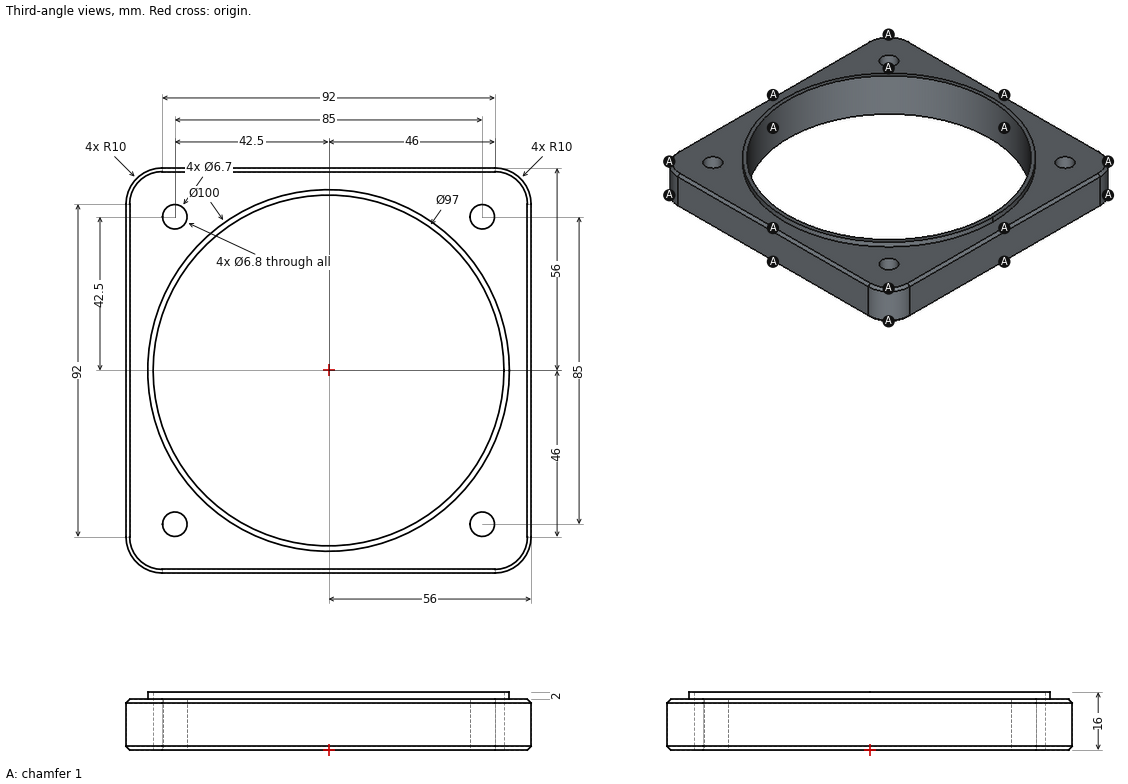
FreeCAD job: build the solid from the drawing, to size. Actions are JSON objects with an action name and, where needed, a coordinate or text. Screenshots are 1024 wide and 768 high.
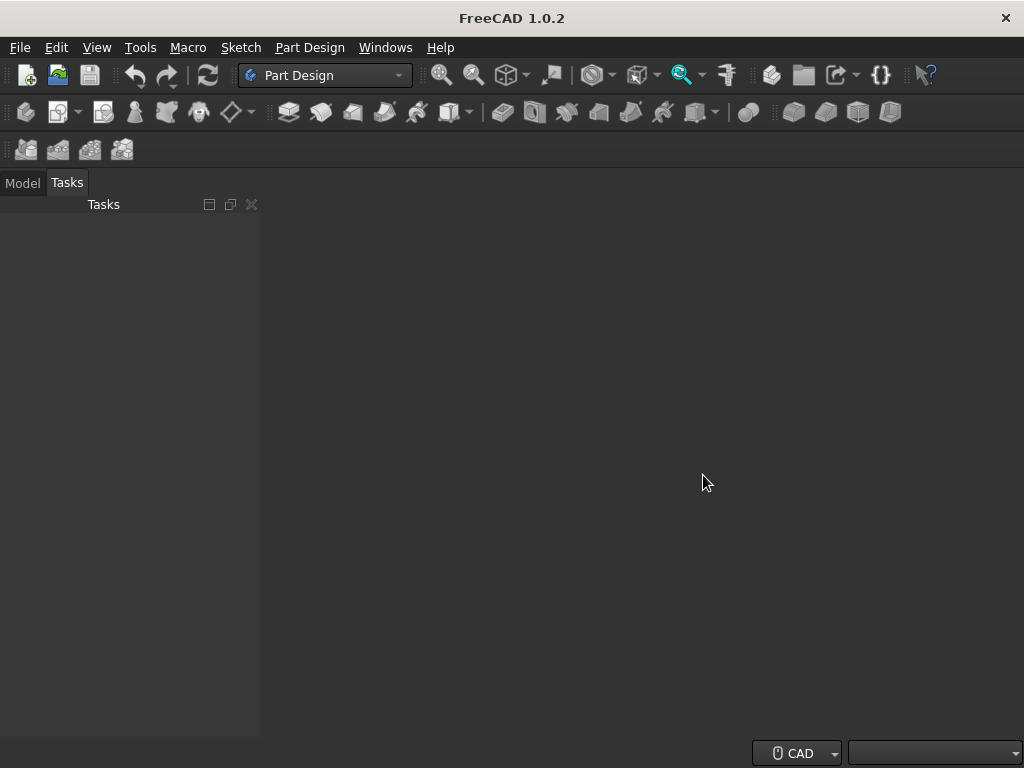
{"action": "left_click", "coordinate": [26, 76]}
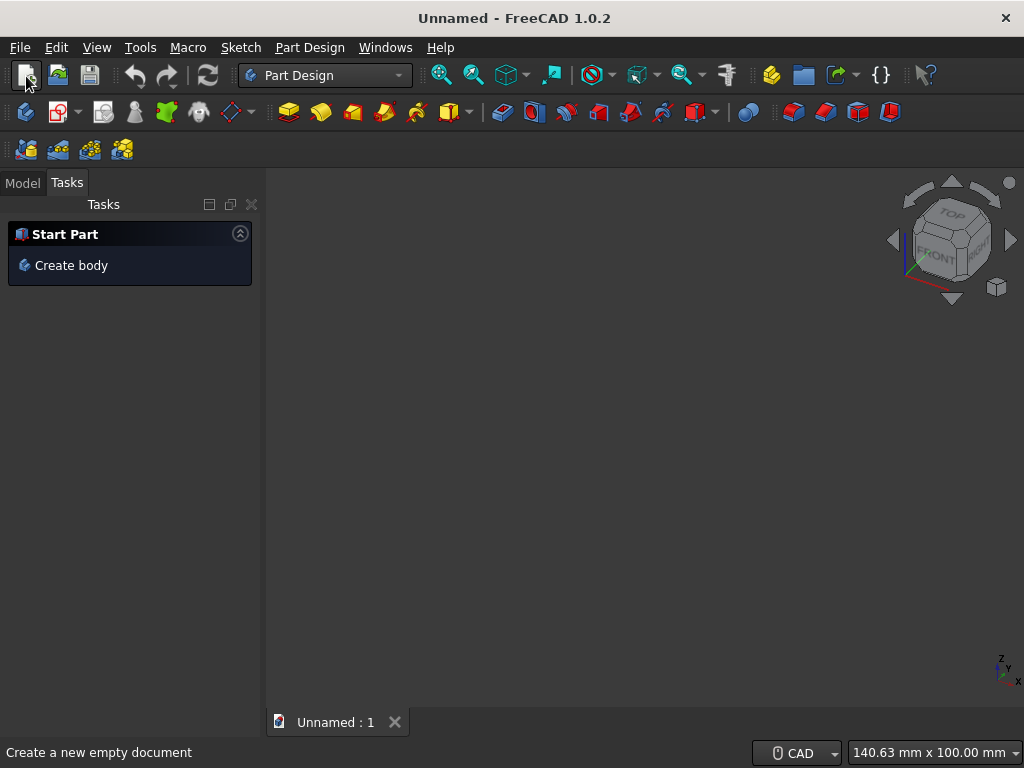
{"action": "left_click", "coordinate": [58, 112]}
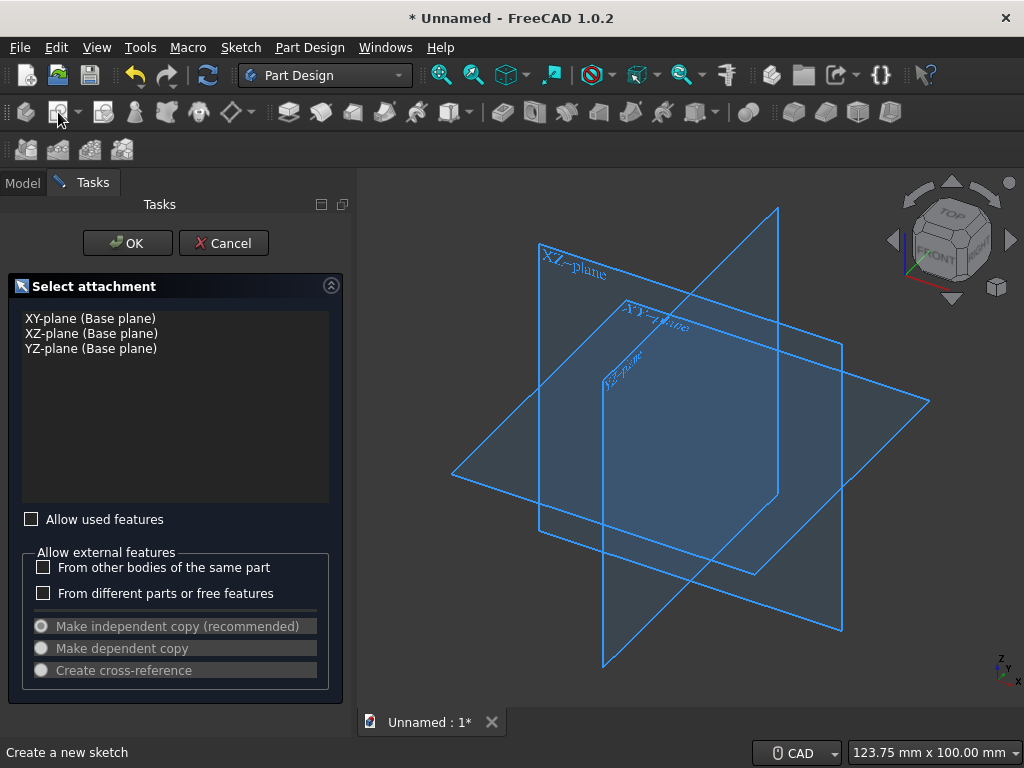
{"action": "left_click", "coordinate": [82, 318]}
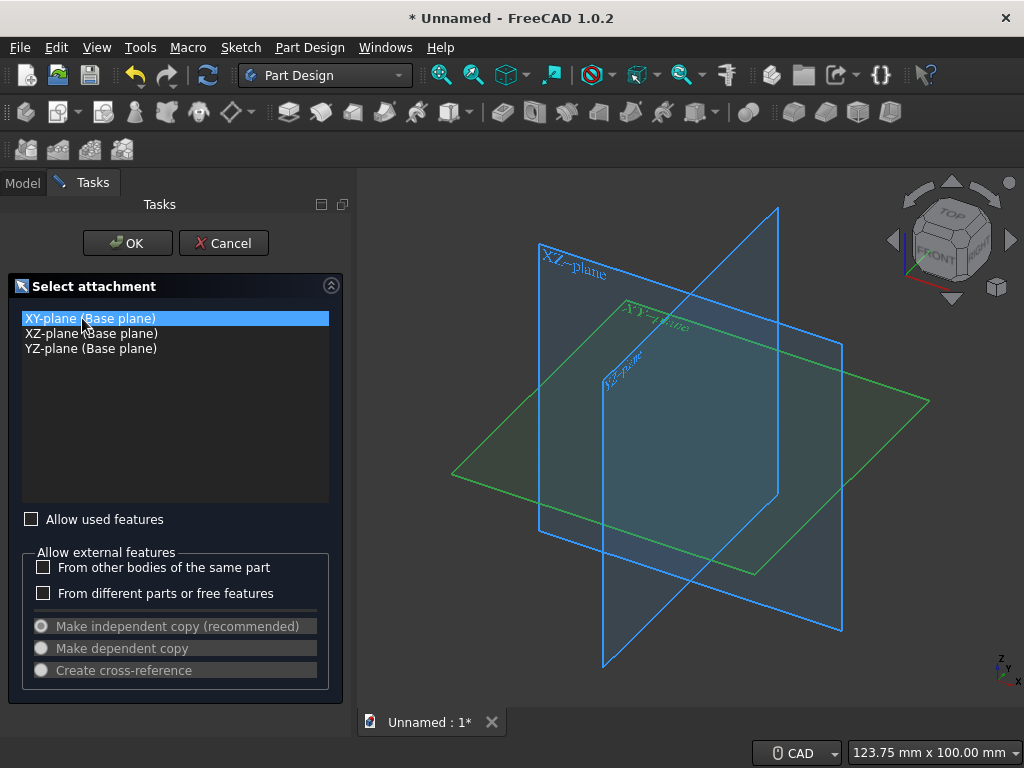
{"action": "left_click", "coordinate": [128, 243]}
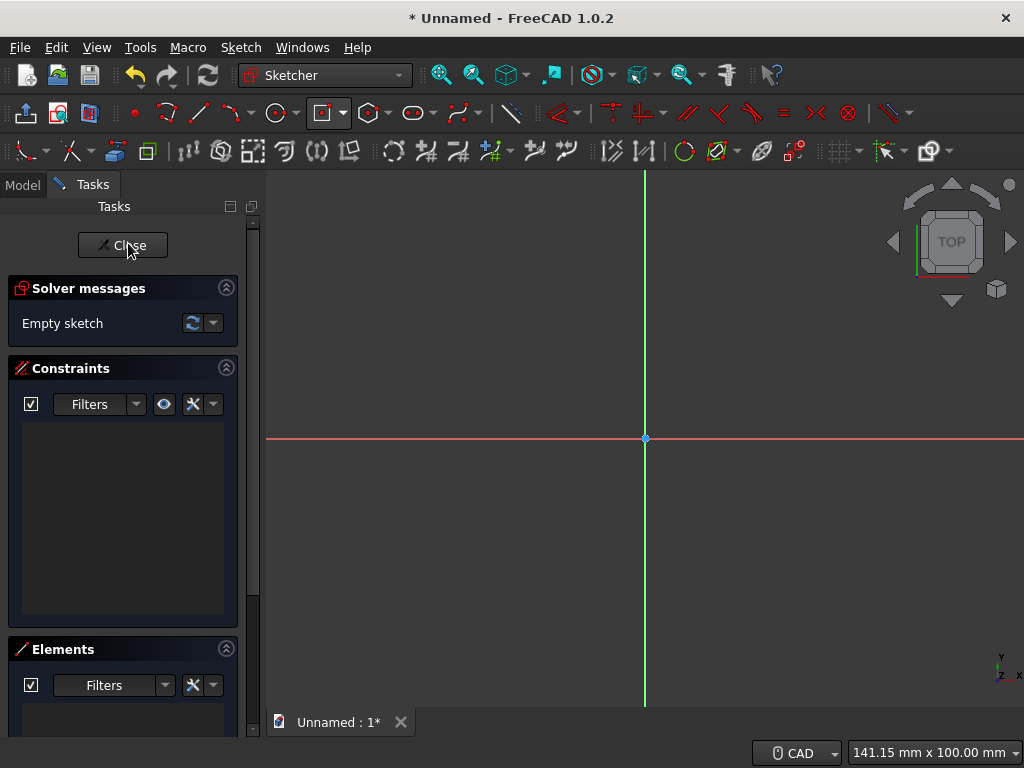
{"action": "scroll", "coordinate": [493, 438], "scroll_direction": "down", "scroll_amount": 3}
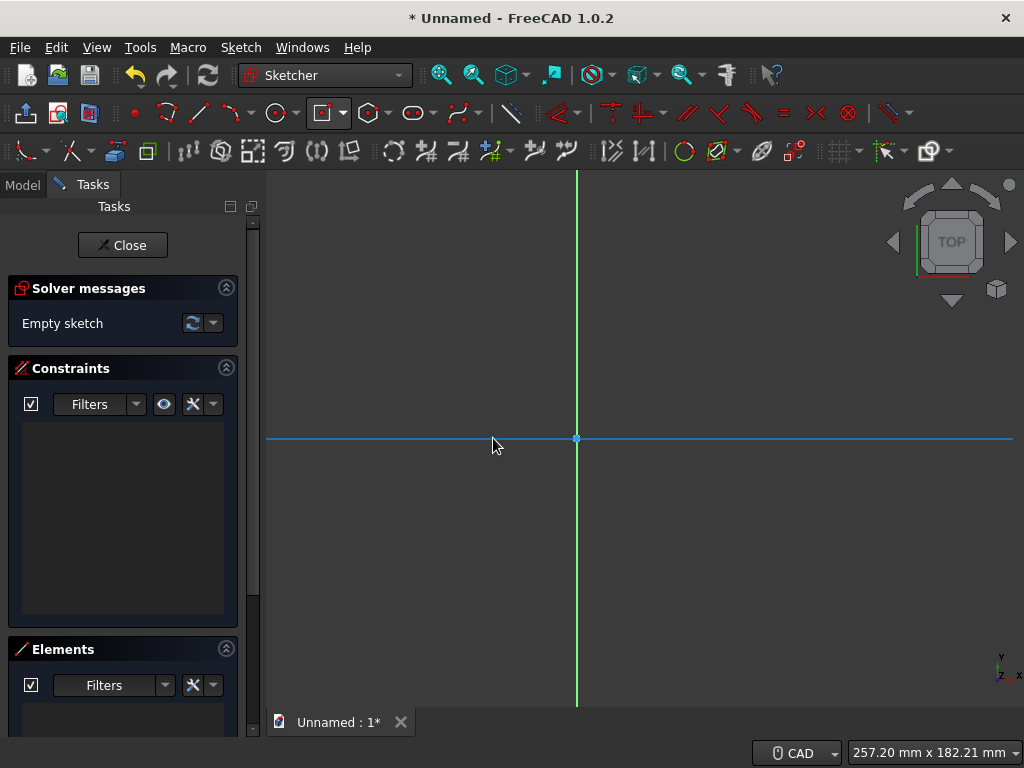
{"action": "left_click", "coordinate": [200, 114]}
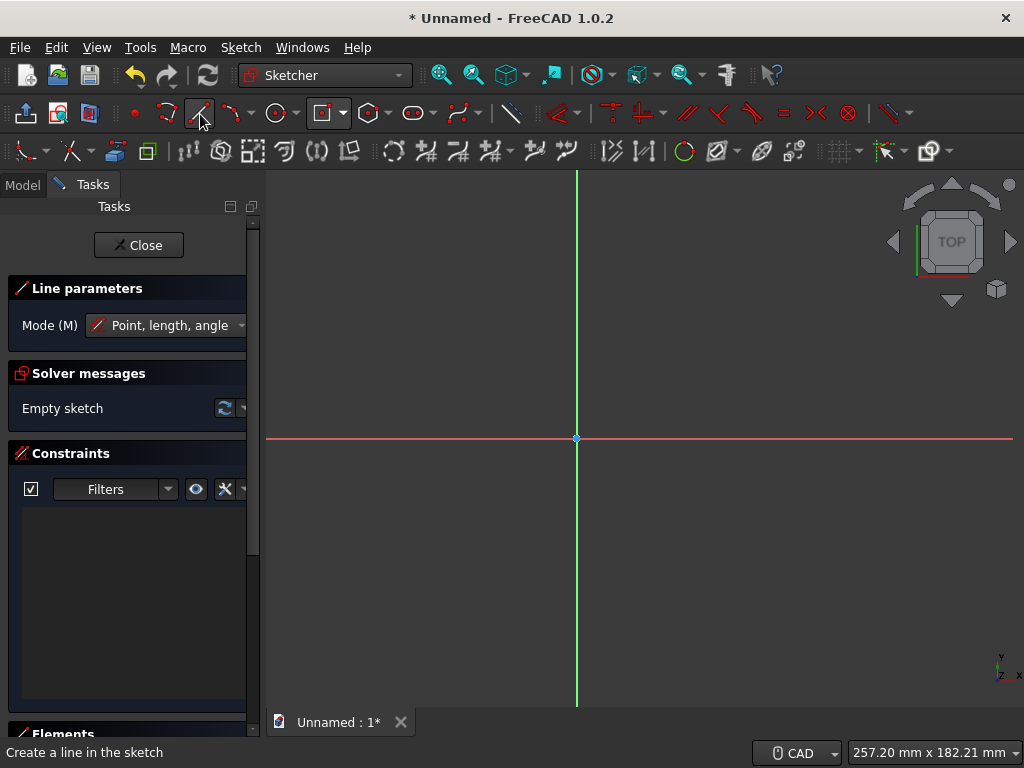
{"action": "left_click", "coordinate": [712, 273]}
{"action": "left_click", "coordinate": [441, 273]}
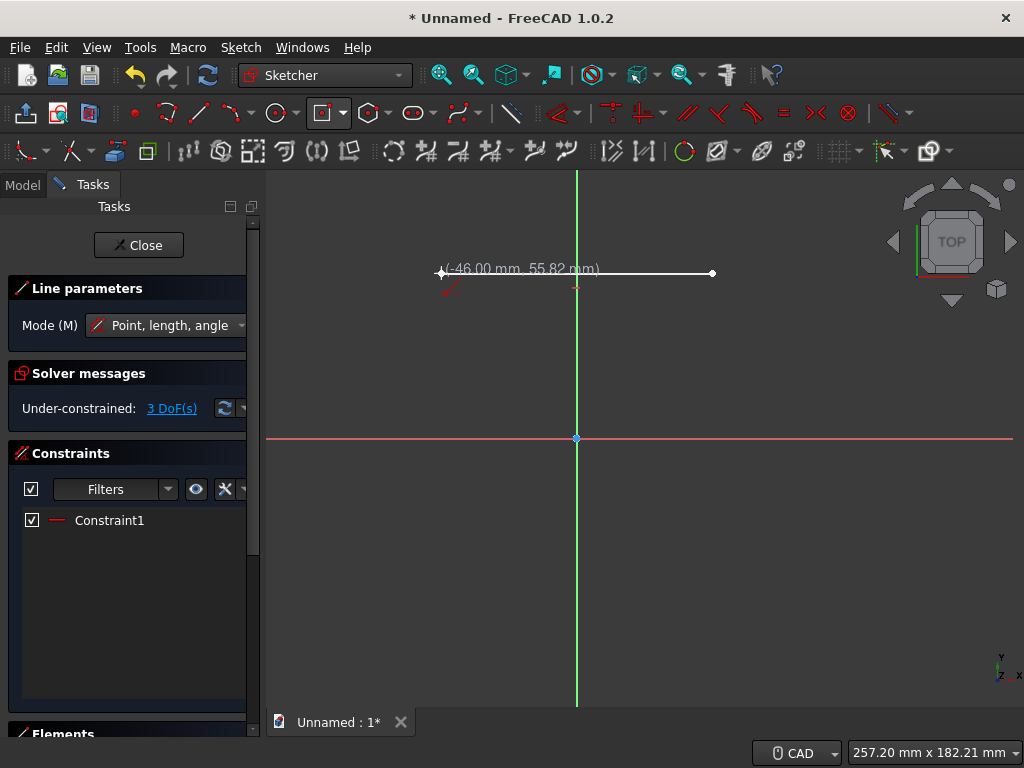
{"action": "left_click", "coordinate": [412, 303]}
{"action": "left_click", "coordinate": [412, 574]}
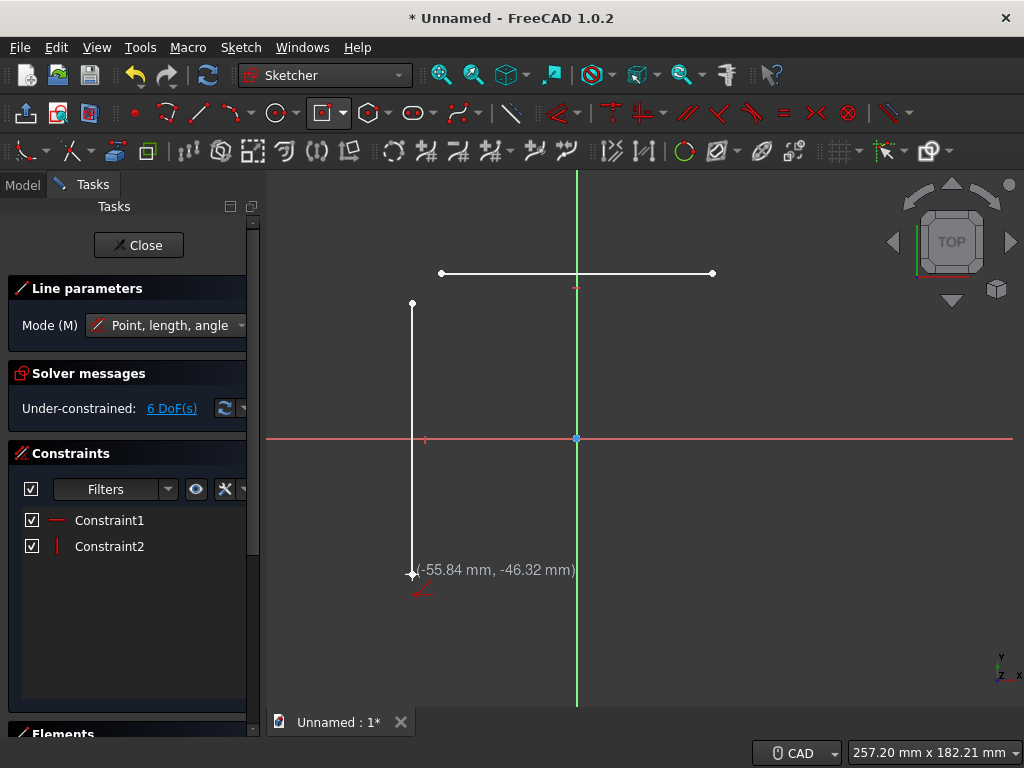
{"action": "left_click", "coordinate": [441, 604]}
{"action": "left_click", "coordinate": [712, 604]}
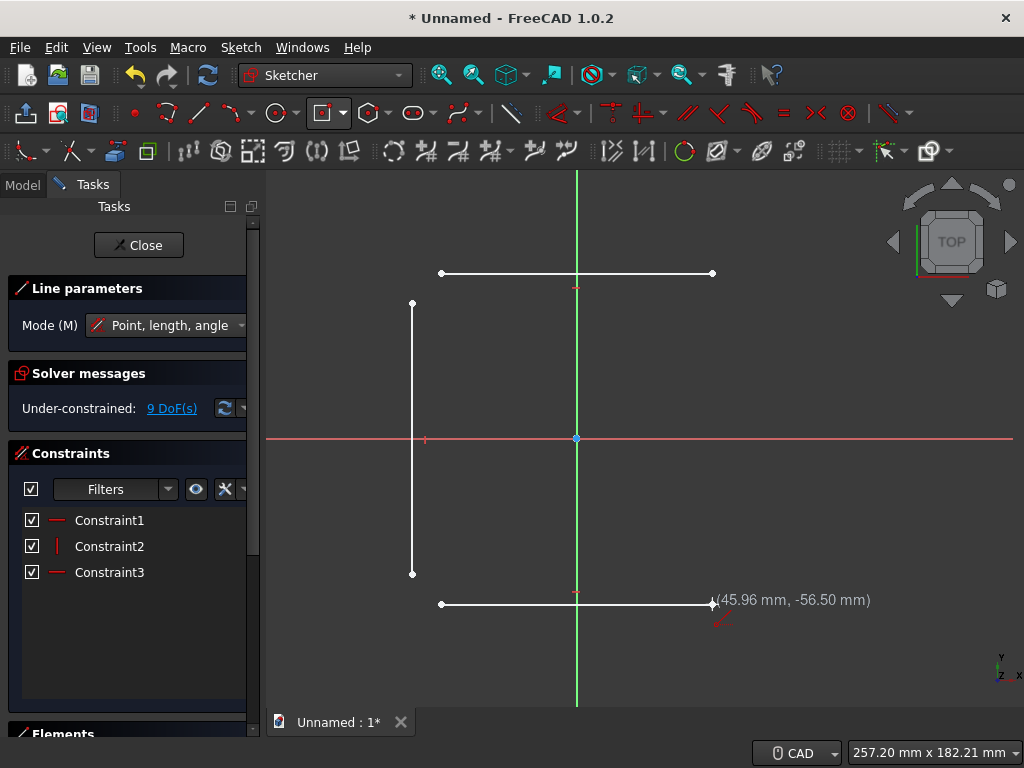
{"action": "left_click", "coordinate": [742, 574]}
{"action": "left_click", "coordinate": [742, 303]}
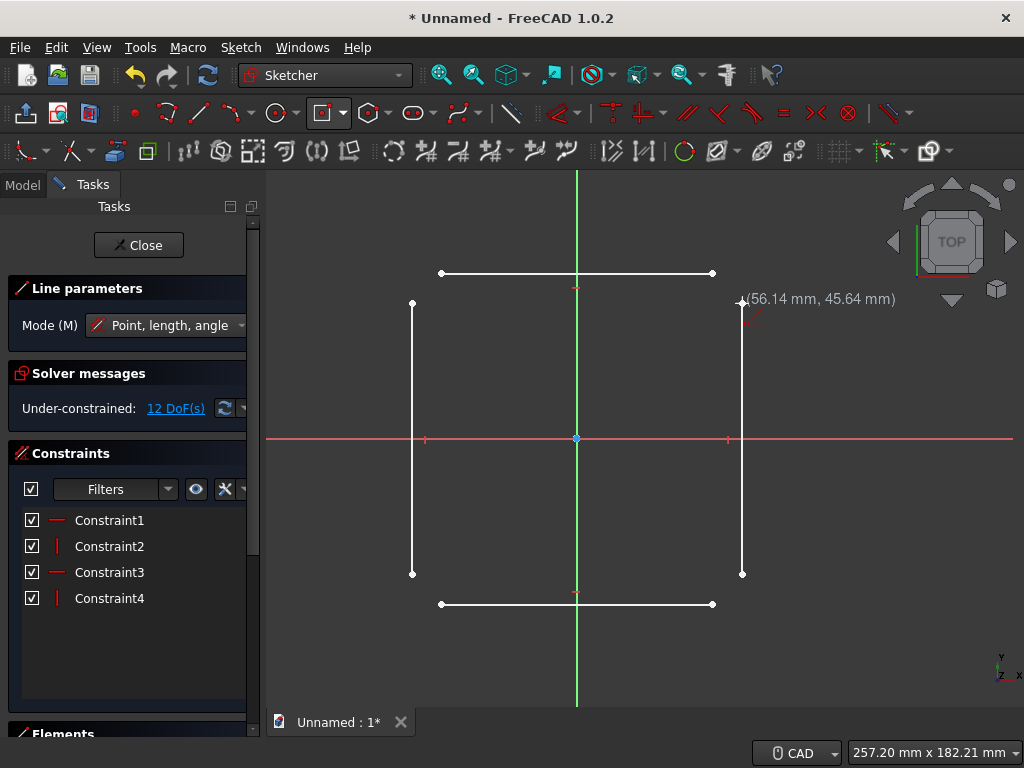
{"action": "left_click", "coordinate": [232, 114]}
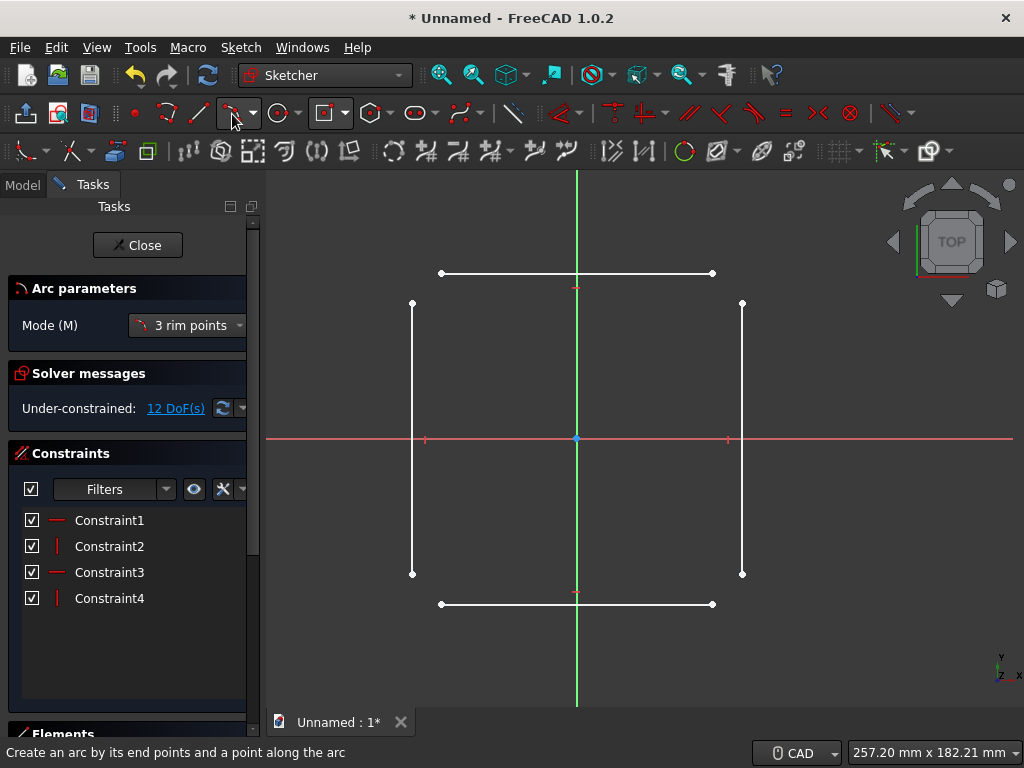
{"action": "left_click", "coordinate": [441, 274]}
{"action": "left_click", "coordinate": [412, 304]}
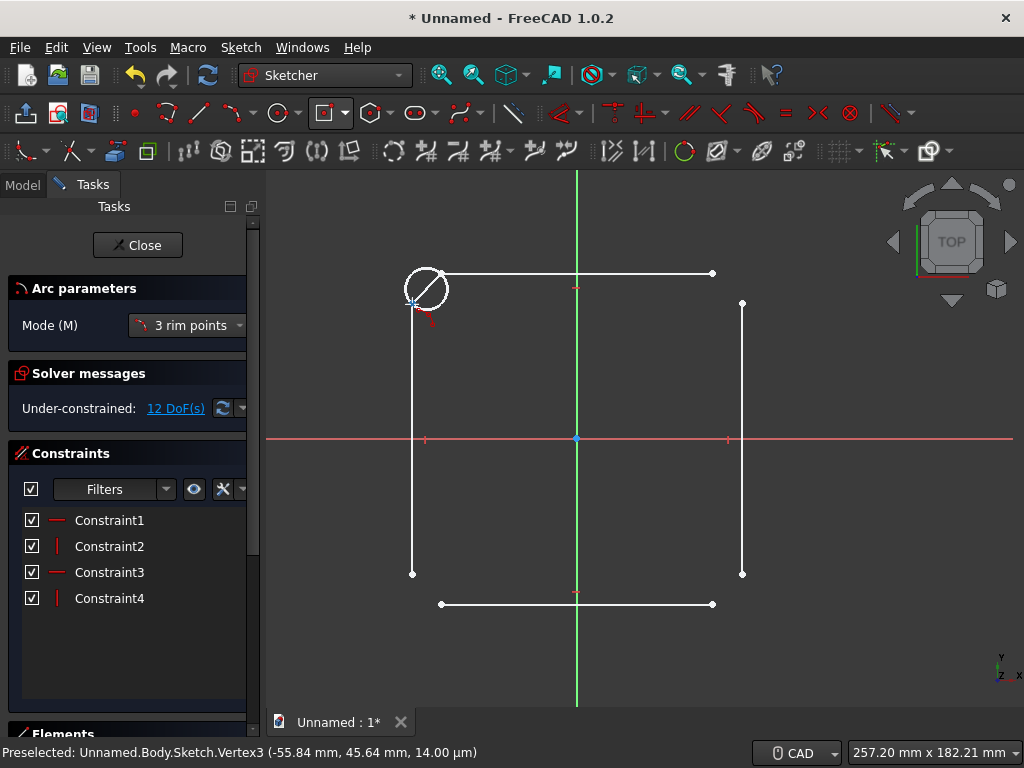
{"action": "scroll", "coordinate": [420, 282], "scroll_direction": "up", "scroll_amount": 4}